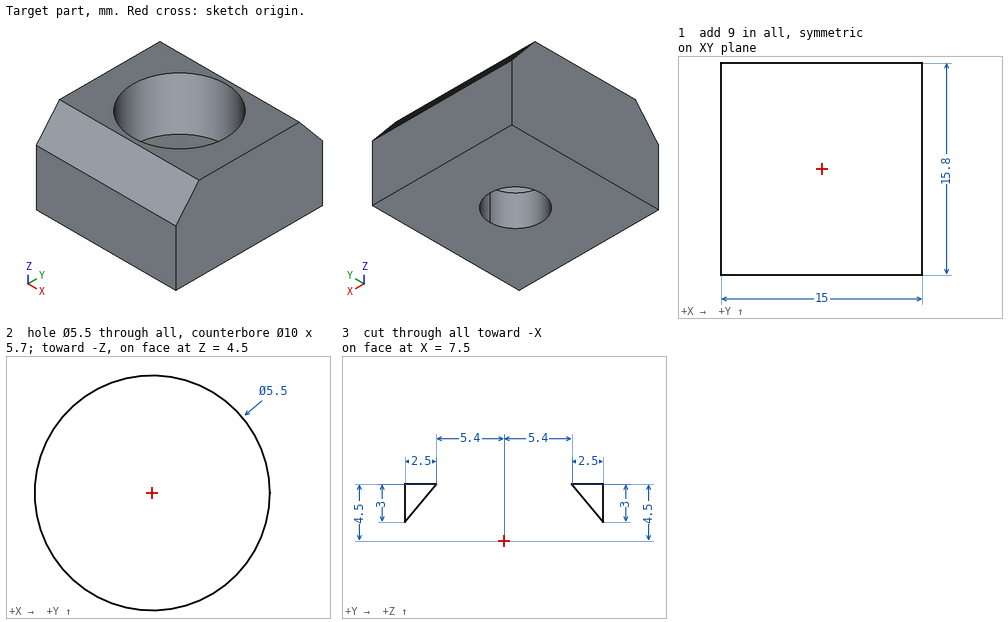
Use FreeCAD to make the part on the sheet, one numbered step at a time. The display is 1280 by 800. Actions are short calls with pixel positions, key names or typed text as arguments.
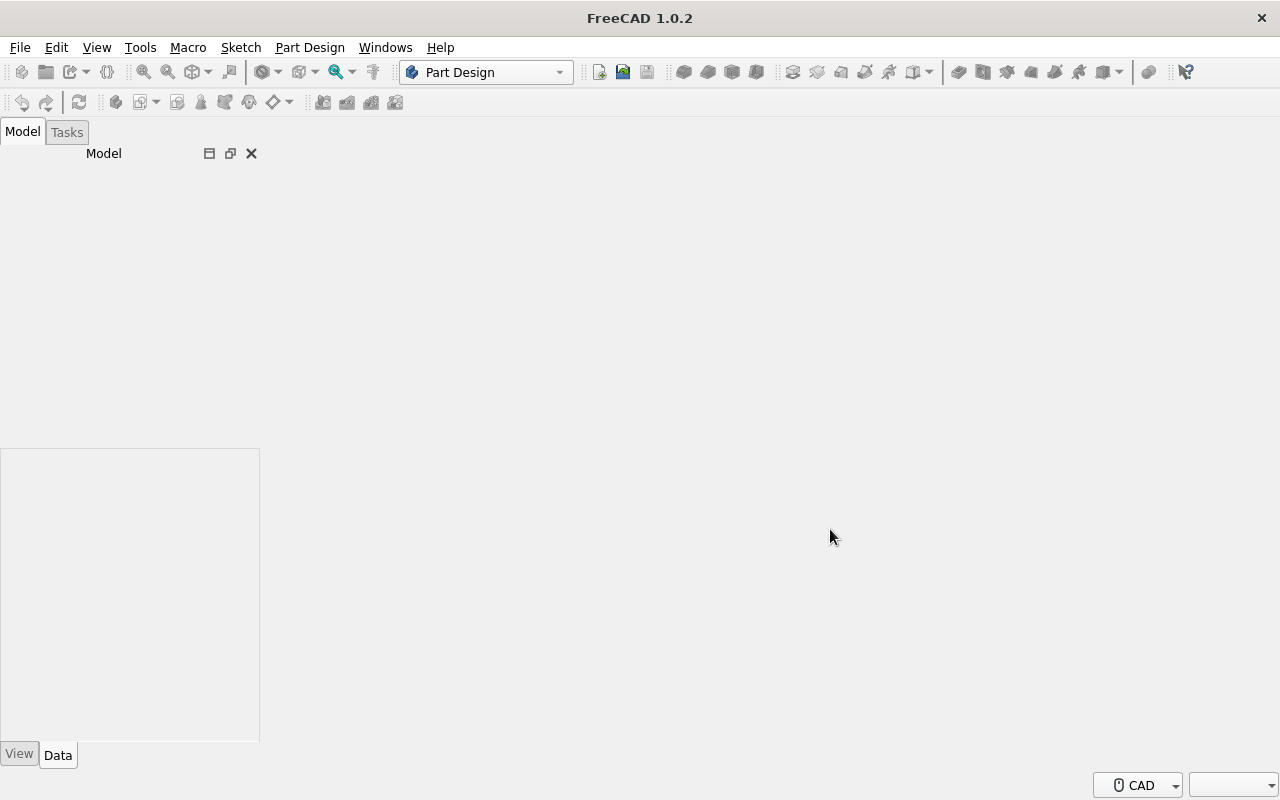
click(600, 72)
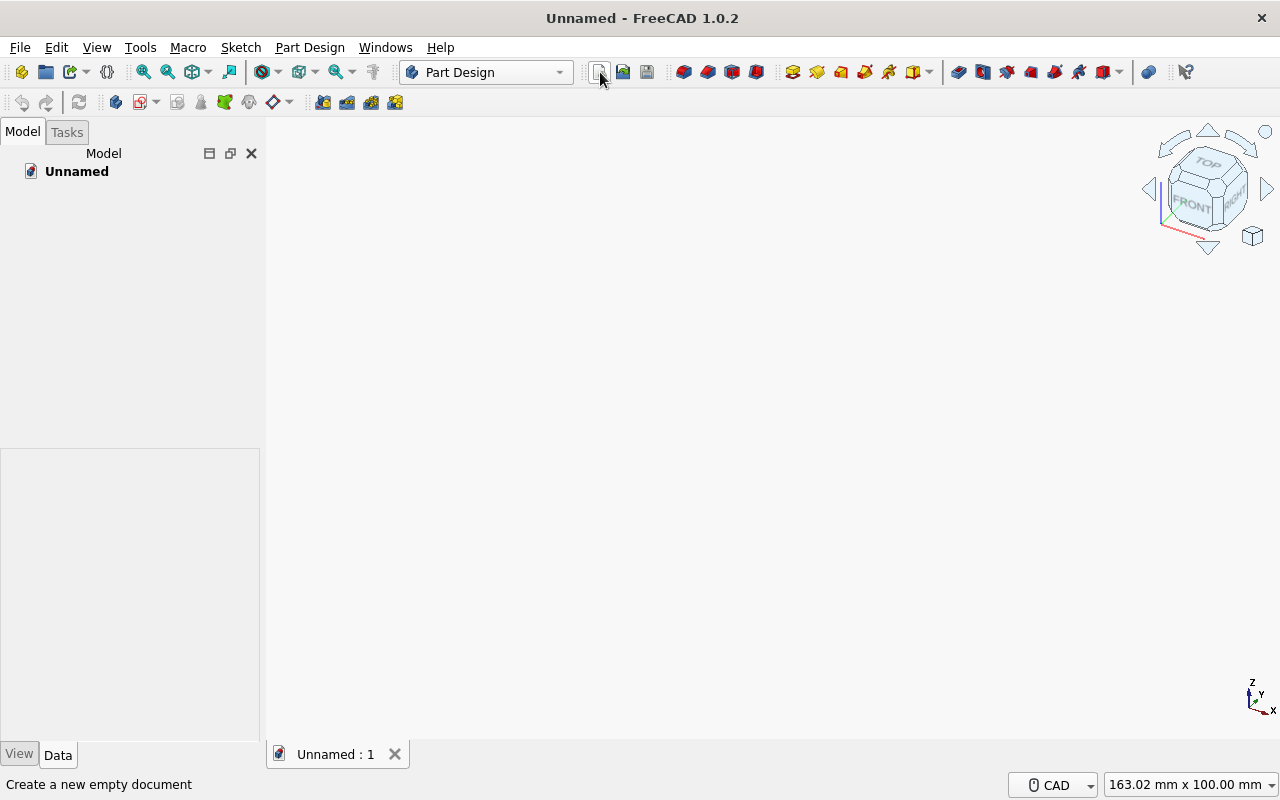
click(140, 102)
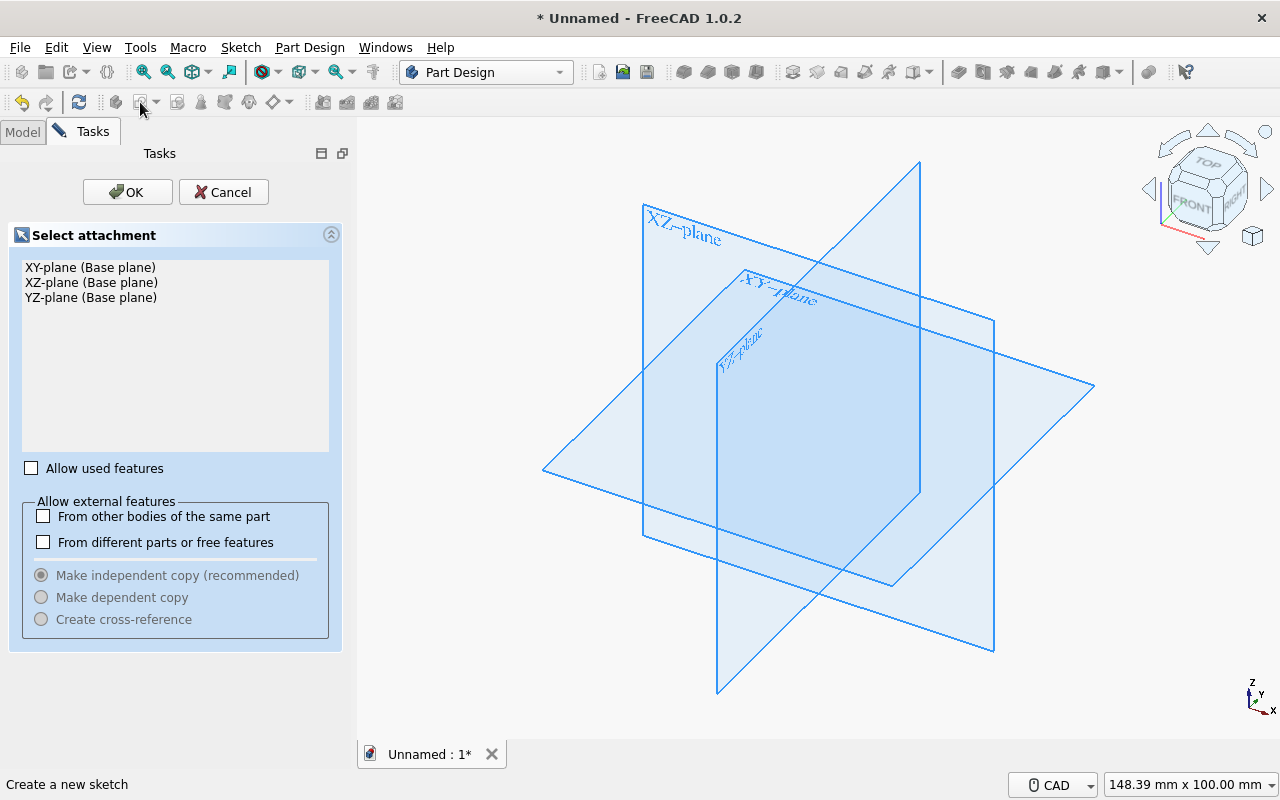
click(82, 268)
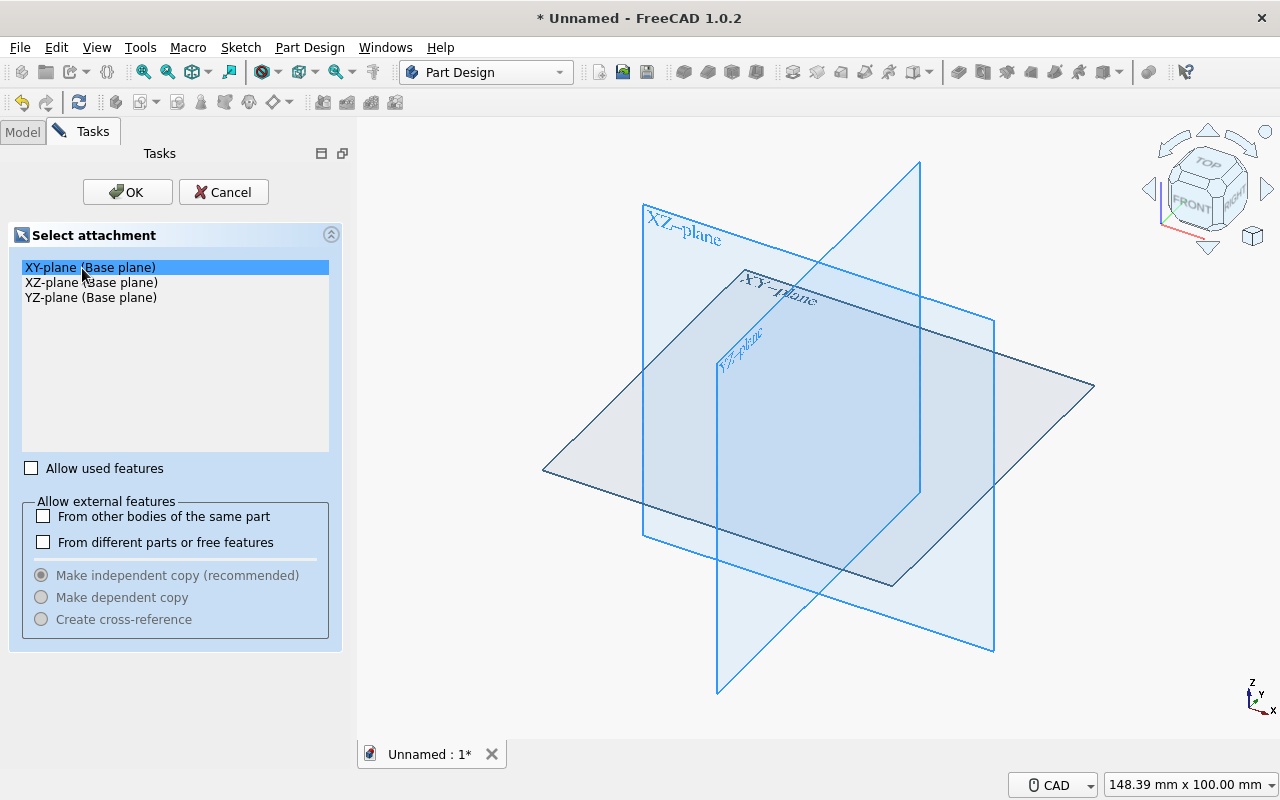
click(128, 192)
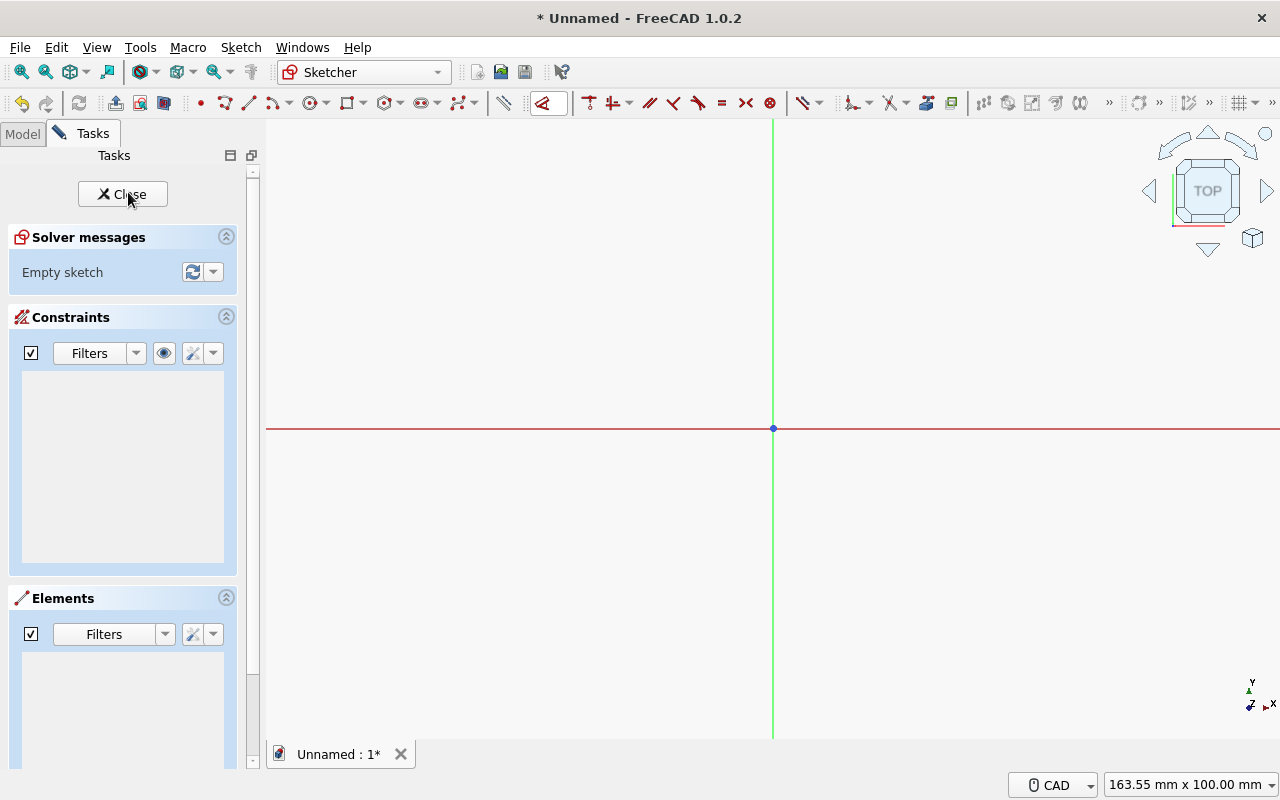
scroll(795, 429, up, 7)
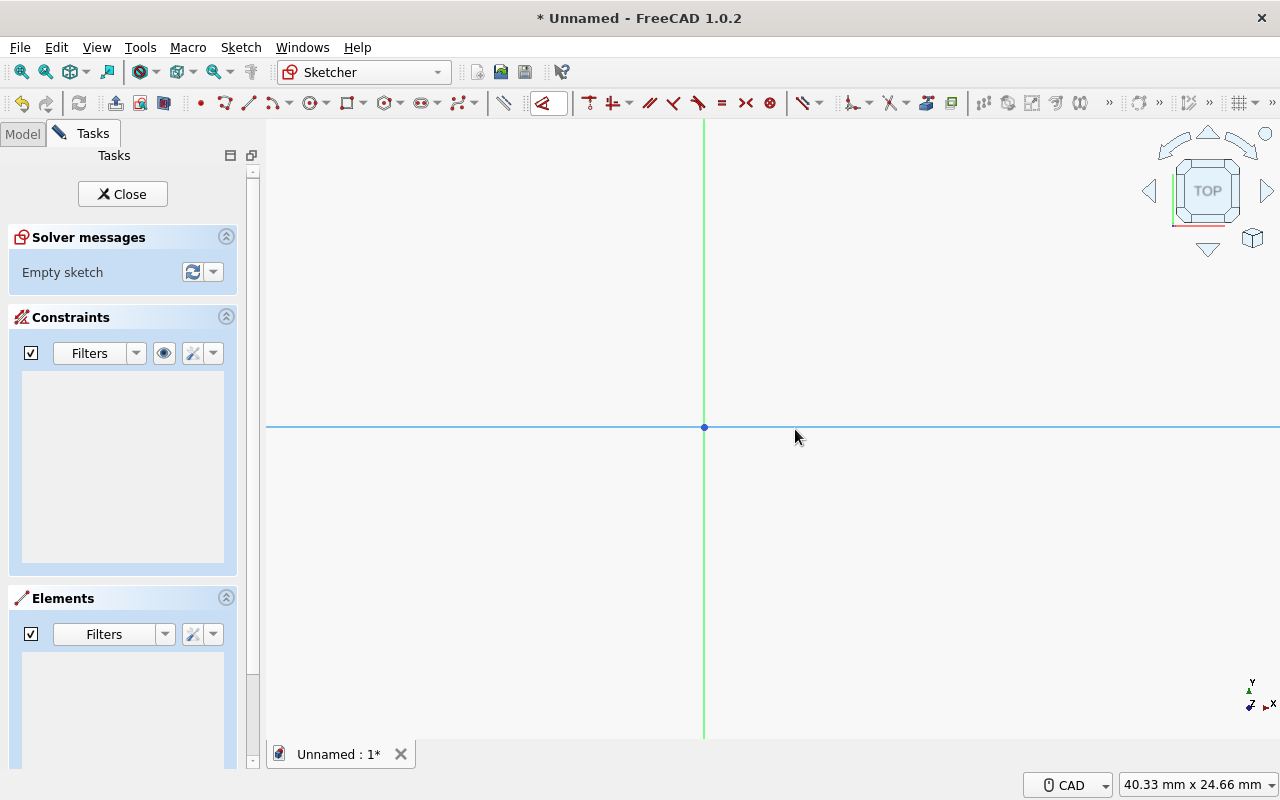
key(g)
key(v)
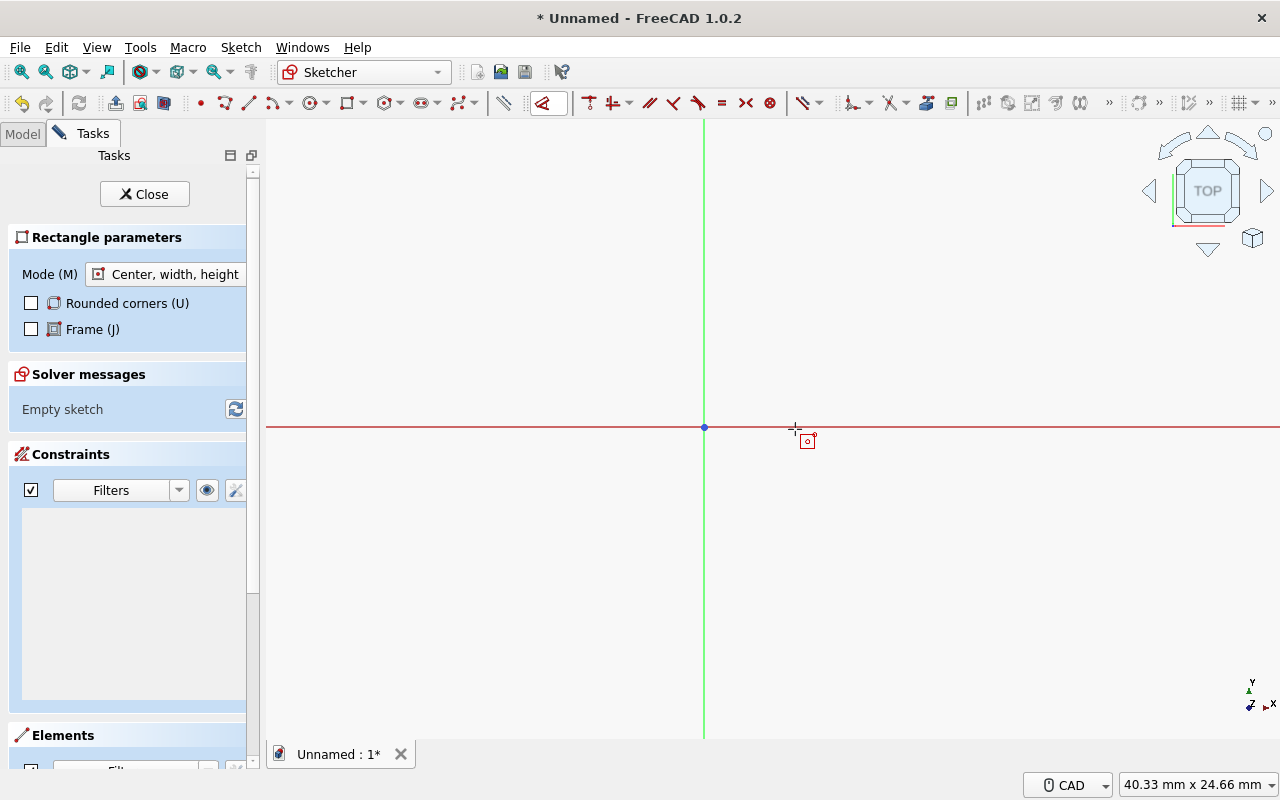
click(704, 427)
click(893, 229)
key(Escape)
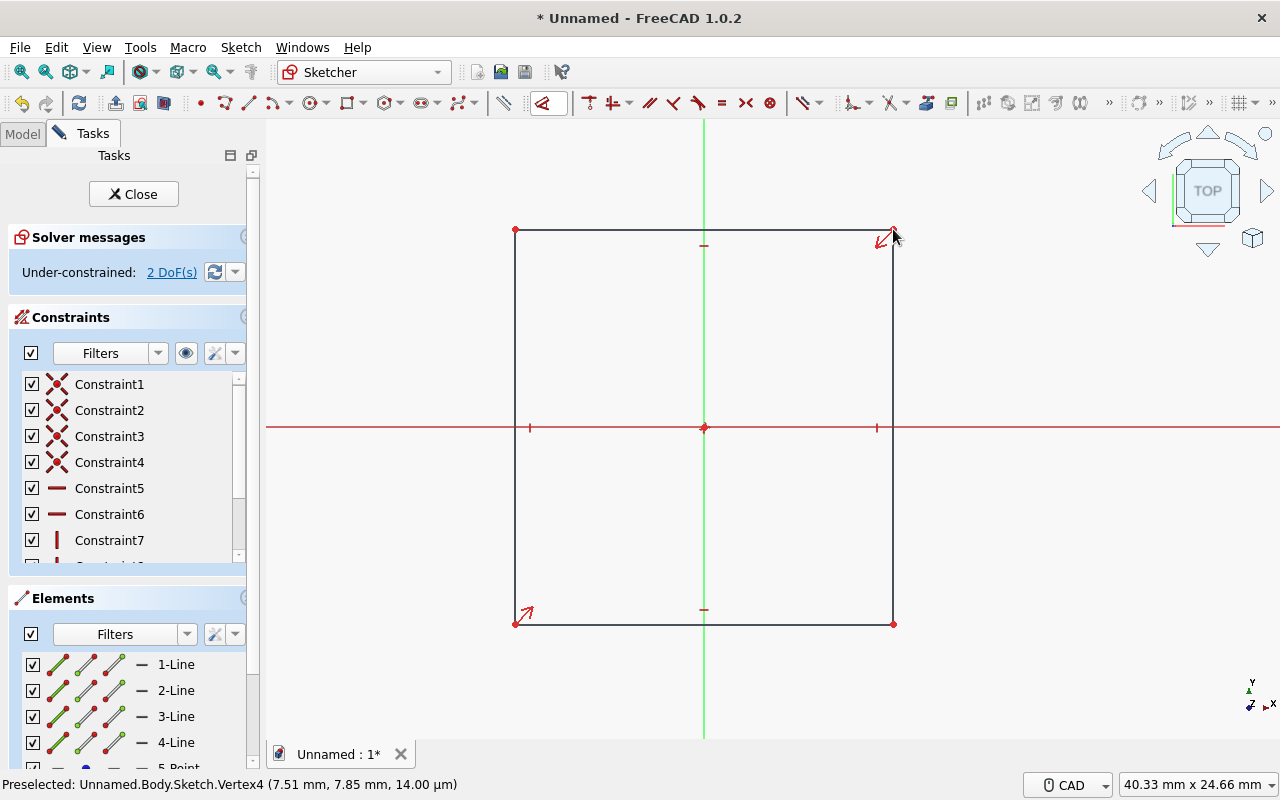
click(629, 625)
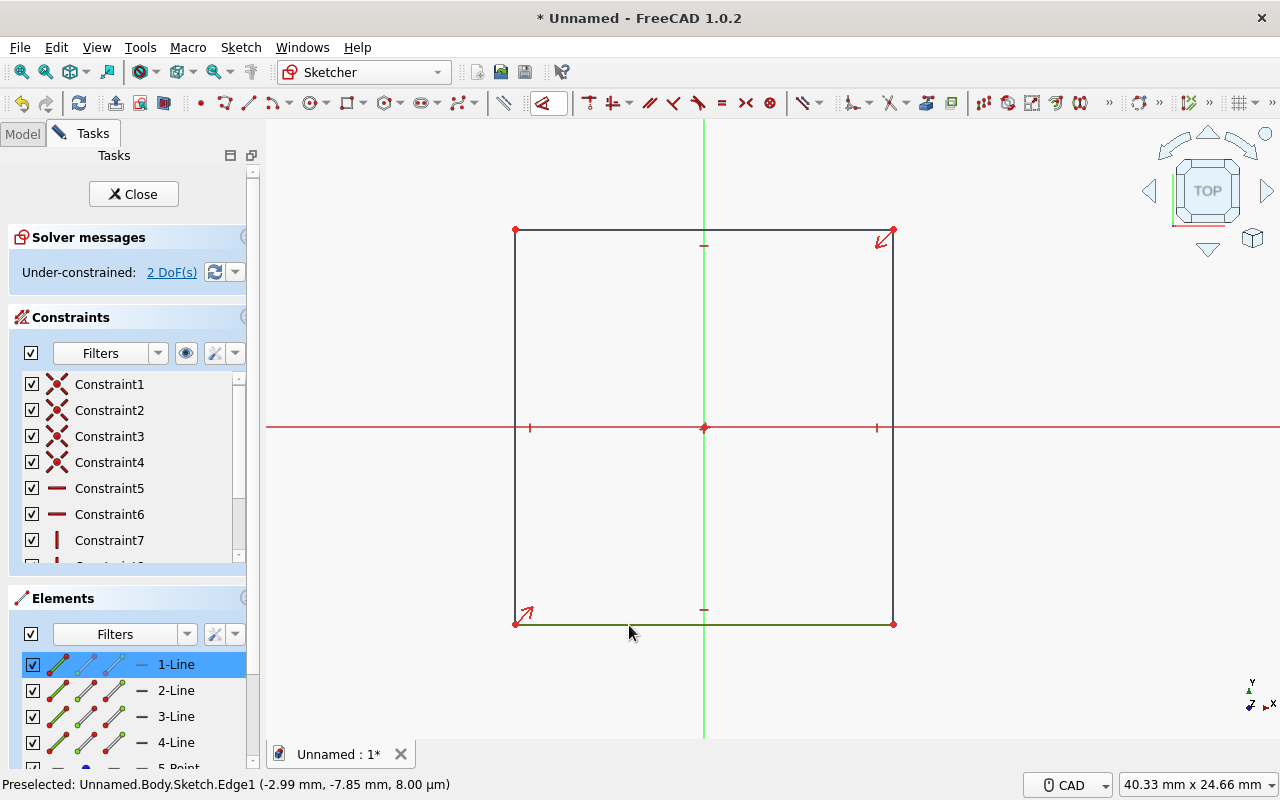
click(562, 104)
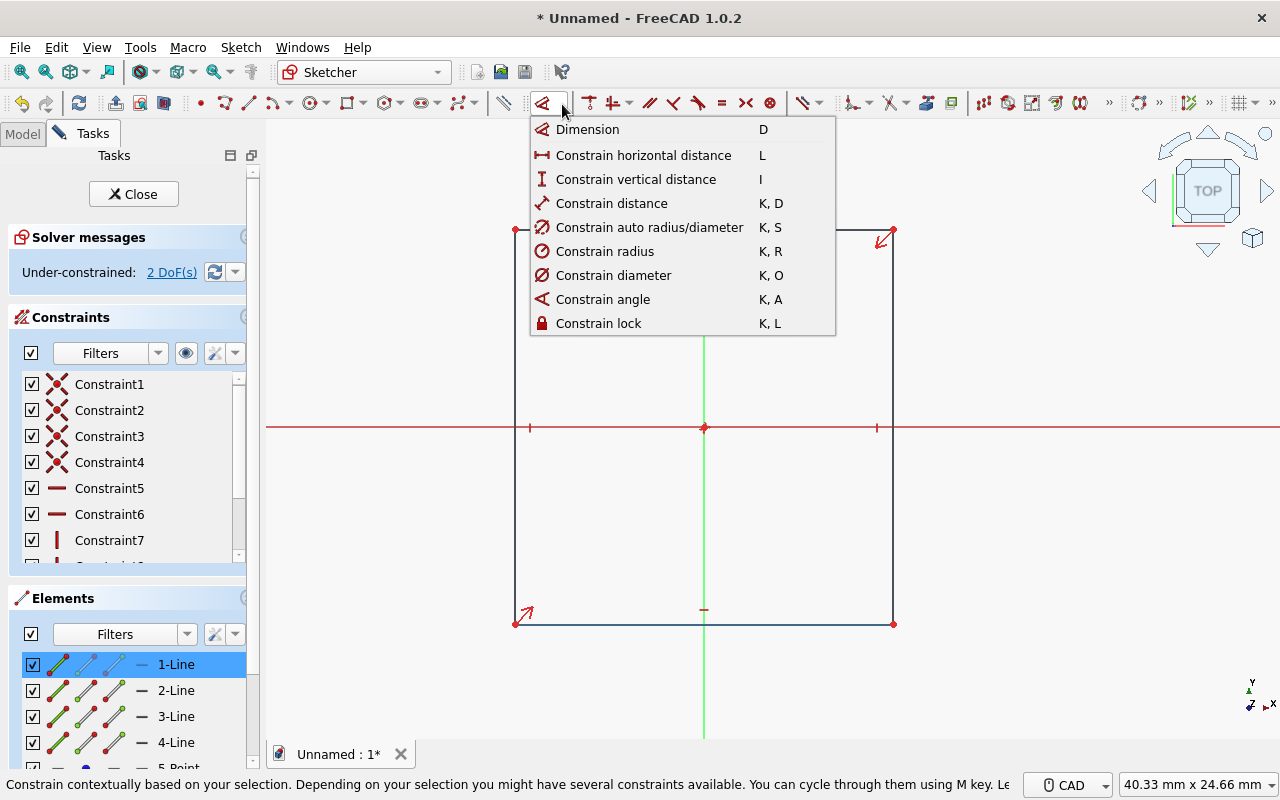
click(683, 155)